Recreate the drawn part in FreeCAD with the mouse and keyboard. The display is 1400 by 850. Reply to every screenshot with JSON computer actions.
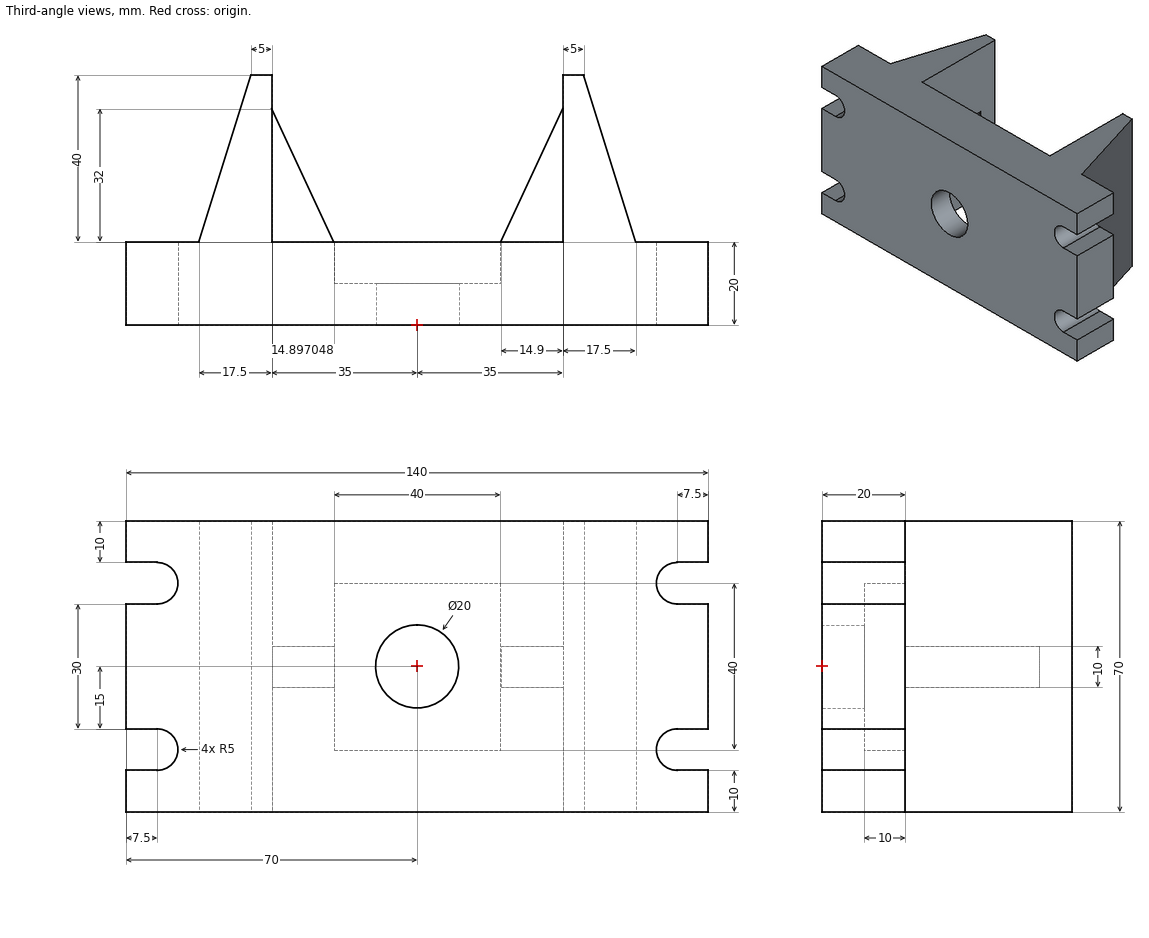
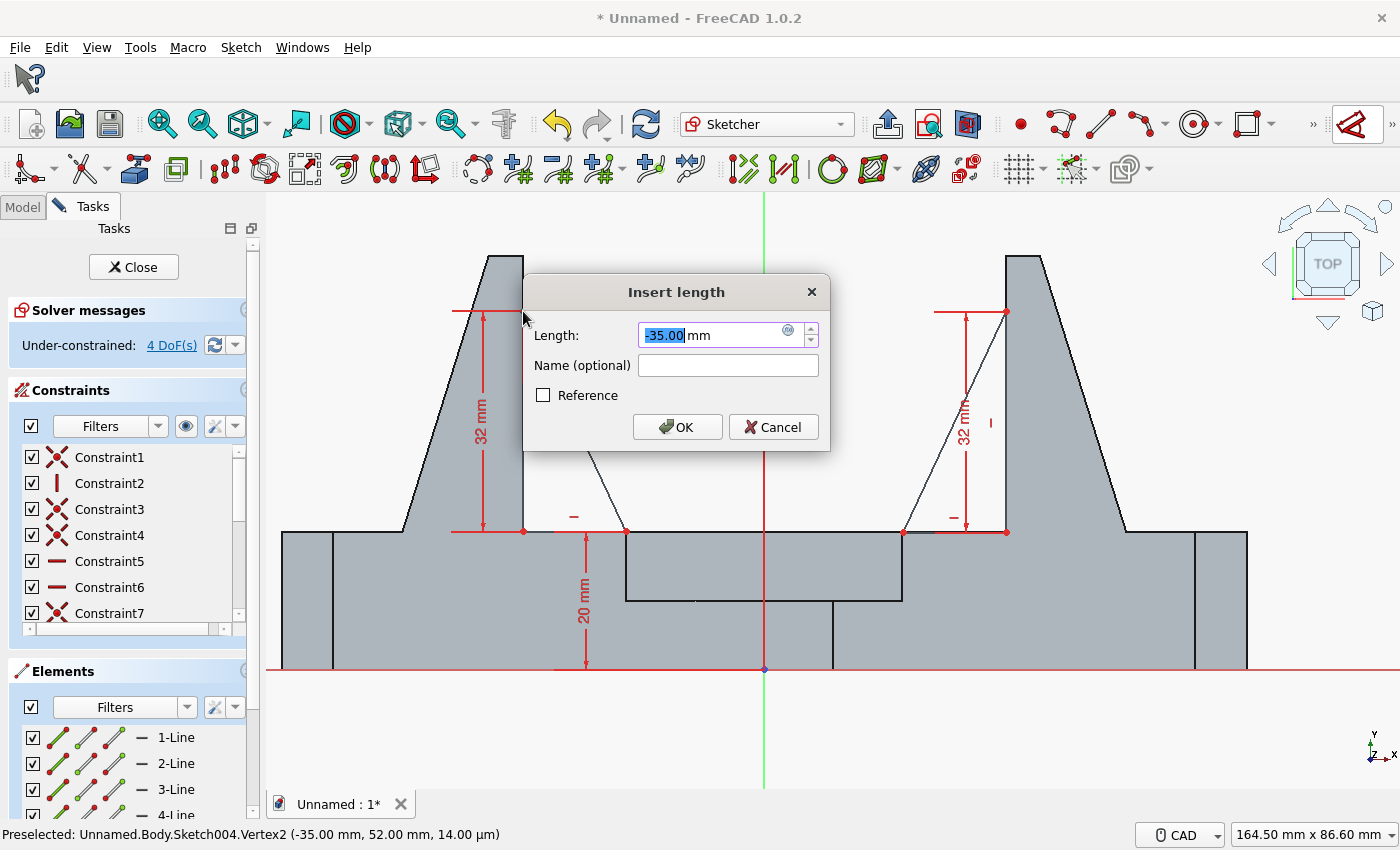
{"action": "type", "text": "-35"}
{"action": "key", "text": "Return"}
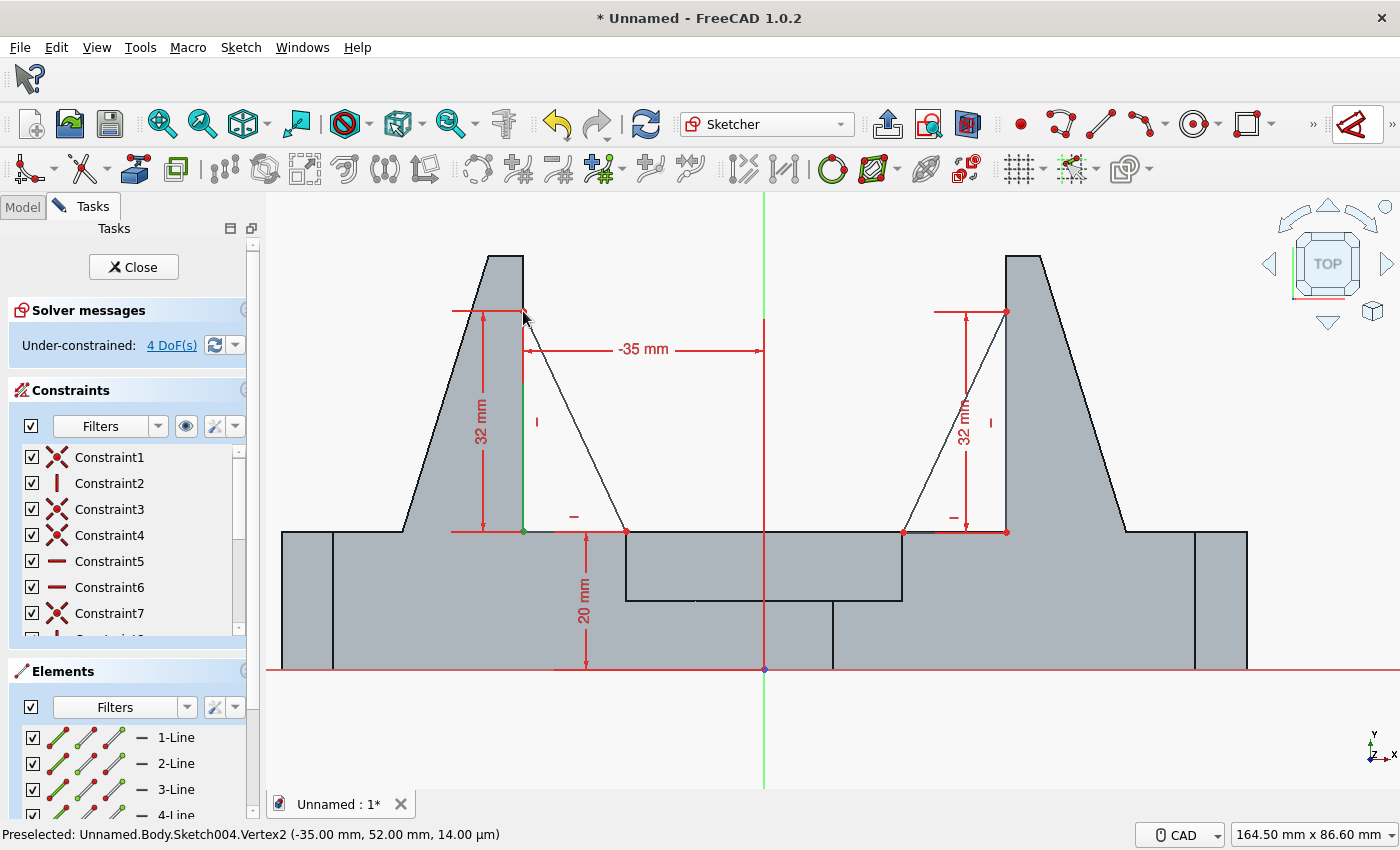
{"action": "left_click", "coordinate": [903, 533]}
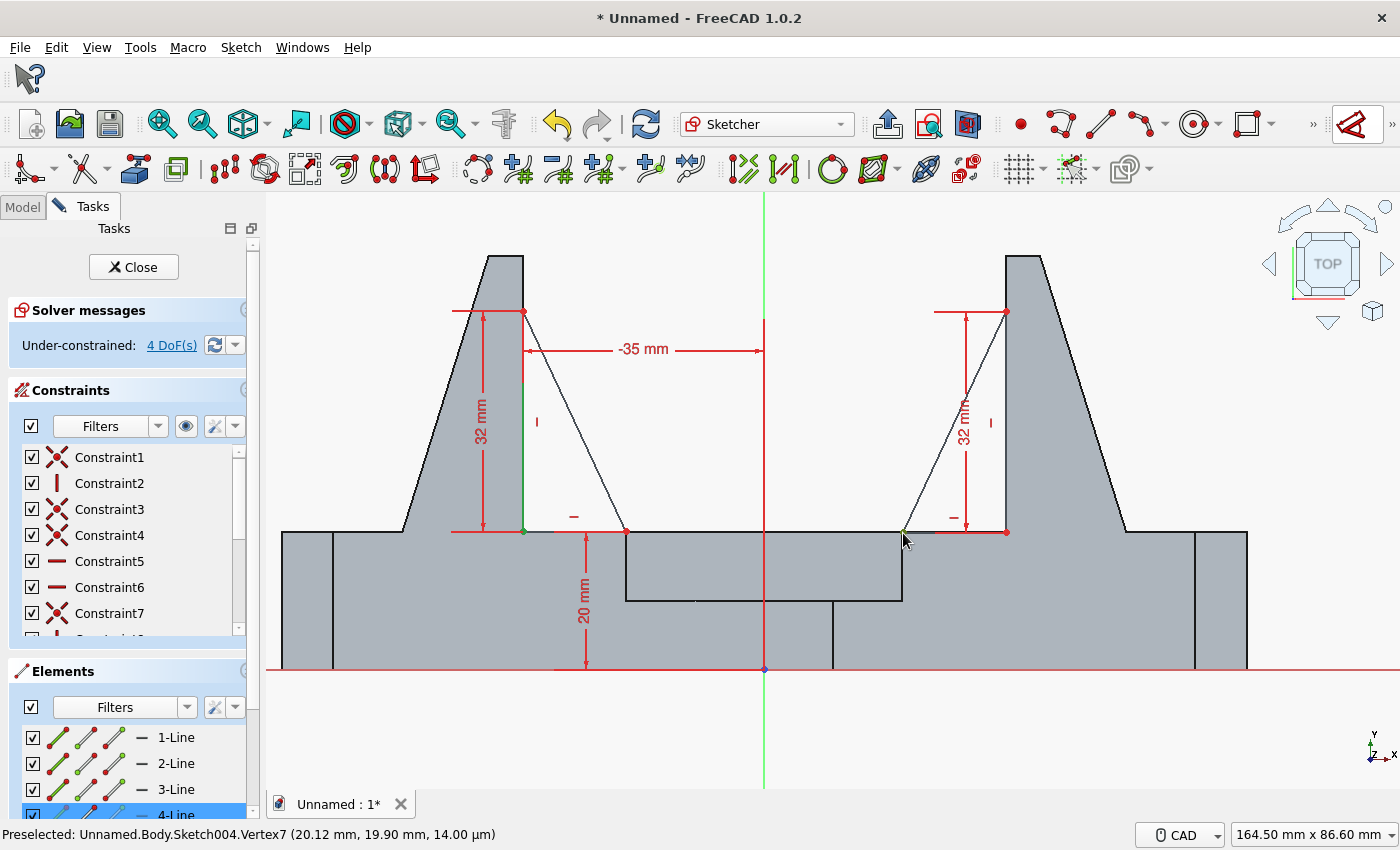
{"action": "key", "text": "i"}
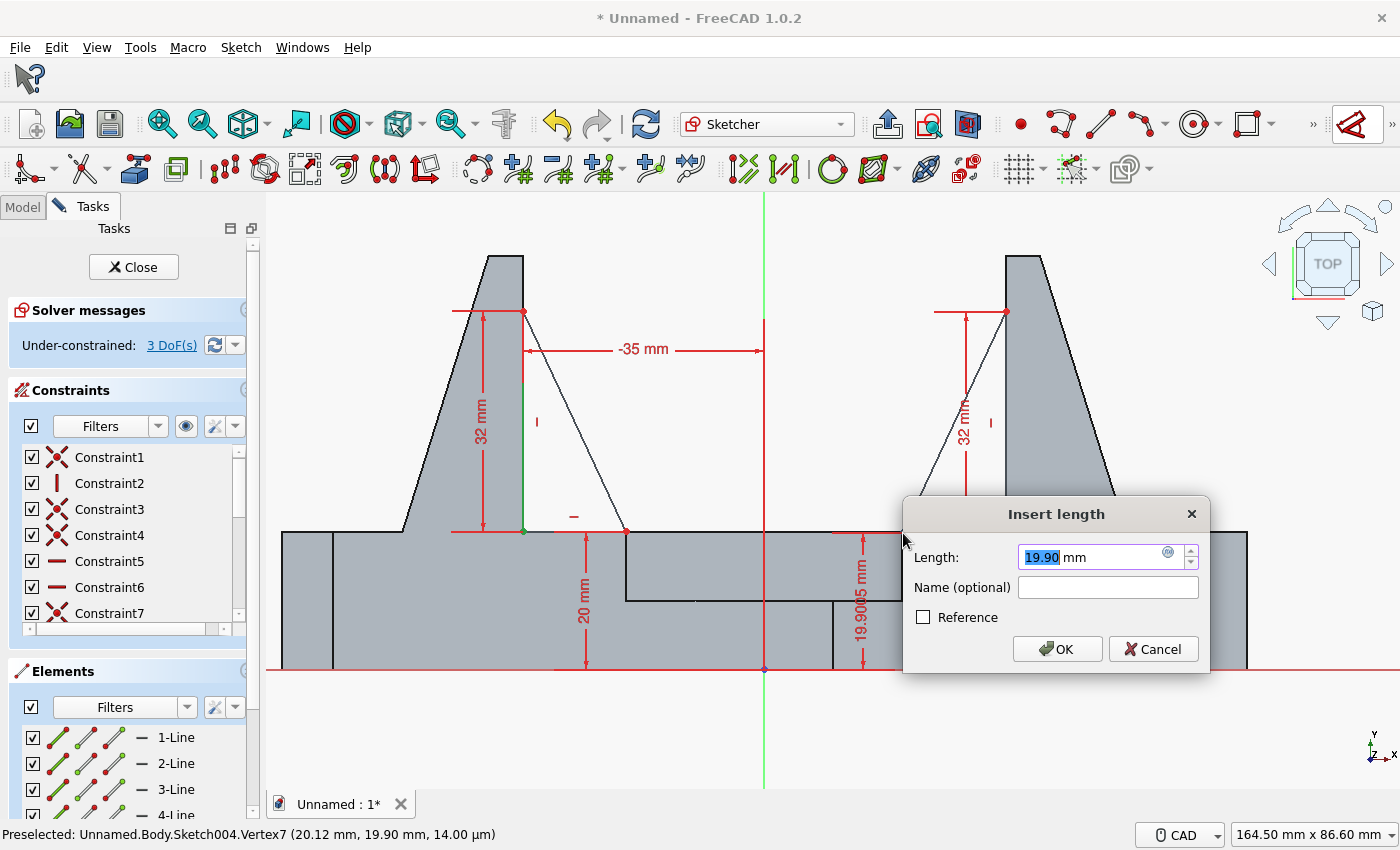
{"action": "type", "text": "20"}
{"action": "key", "text": "Return"}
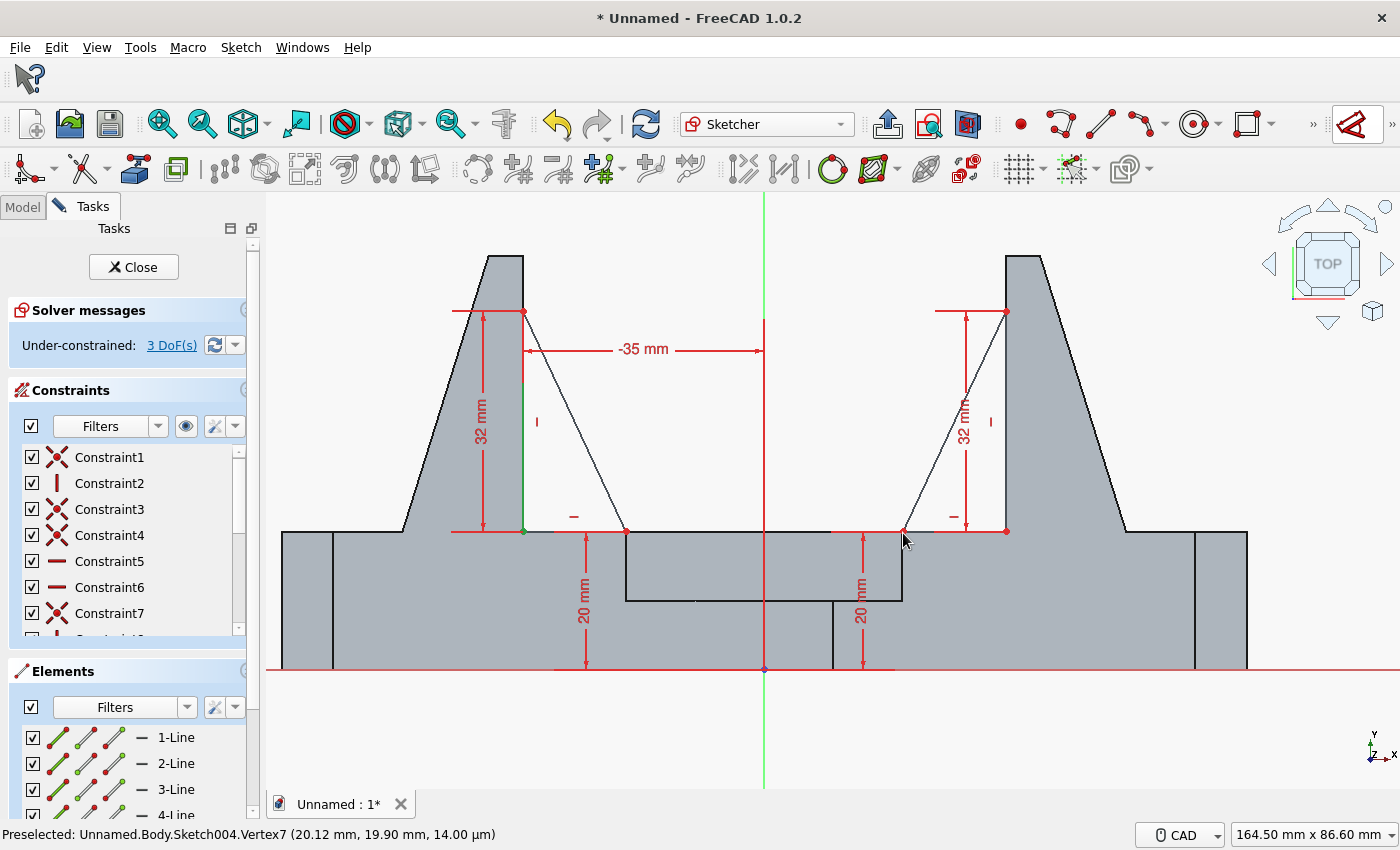
{"action": "left_click", "coordinate": [1006, 532]}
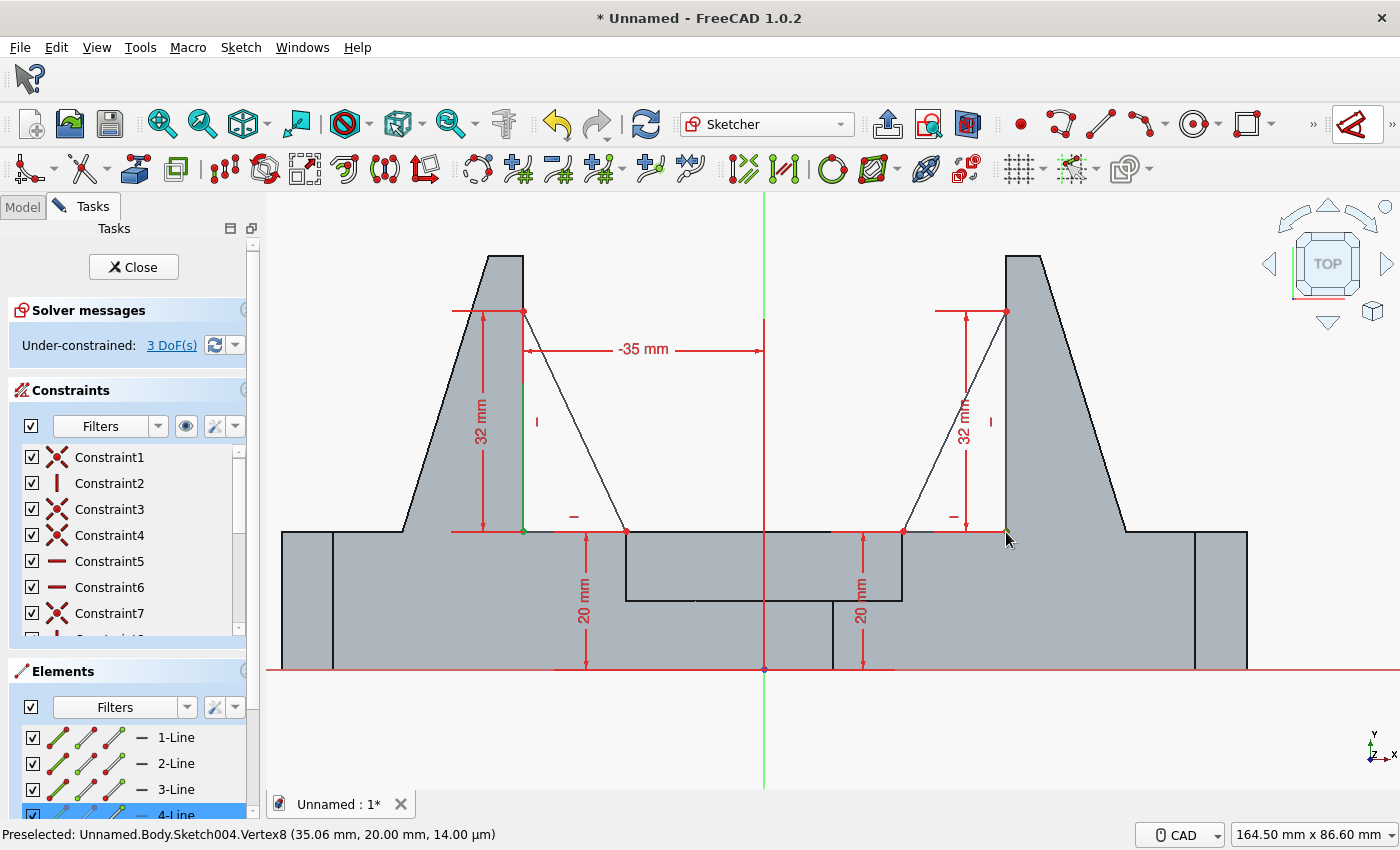
{"action": "left_click", "coordinate": [1378, 124]}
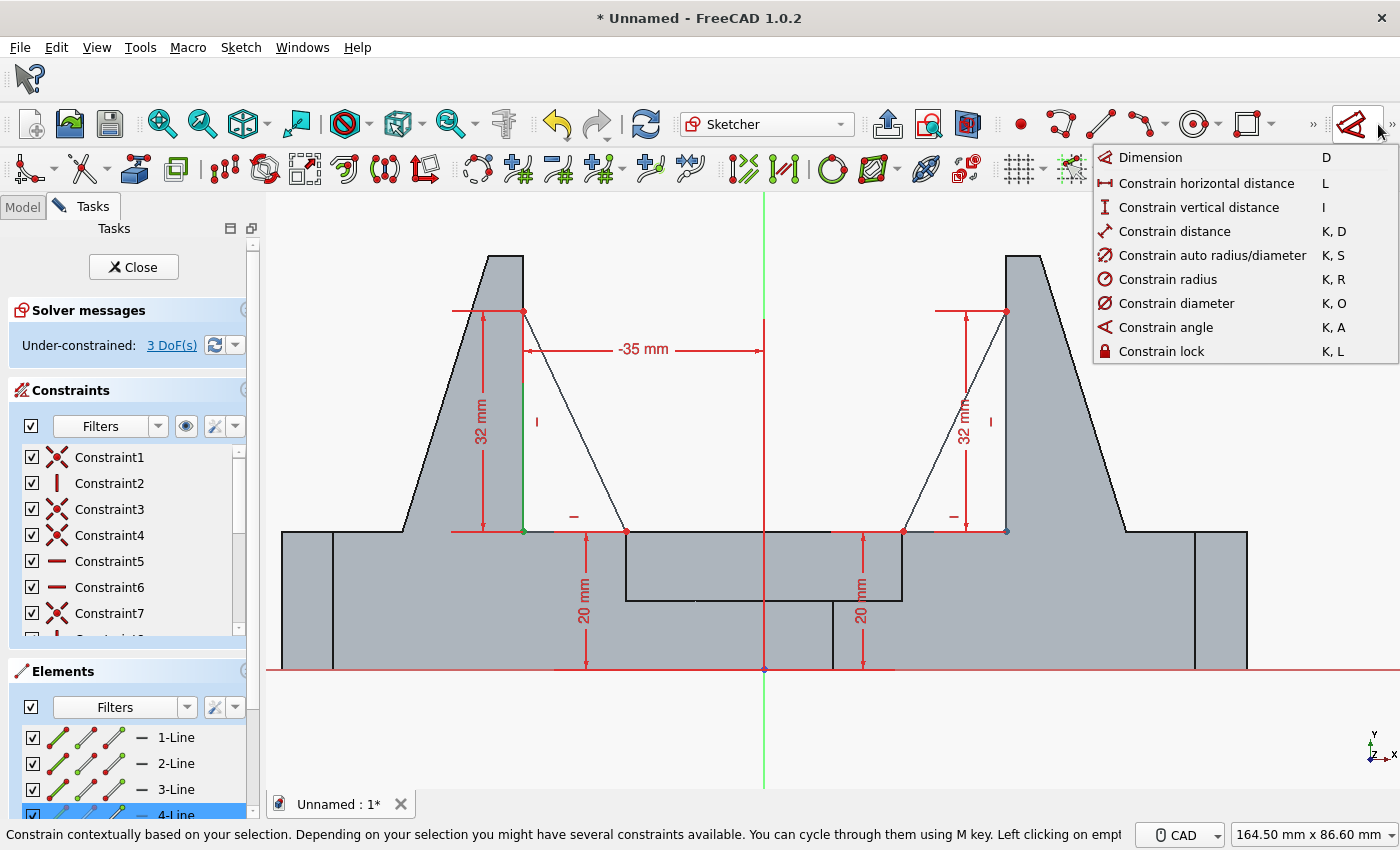
{"action": "left_click", "coordinate": [1246, 183]}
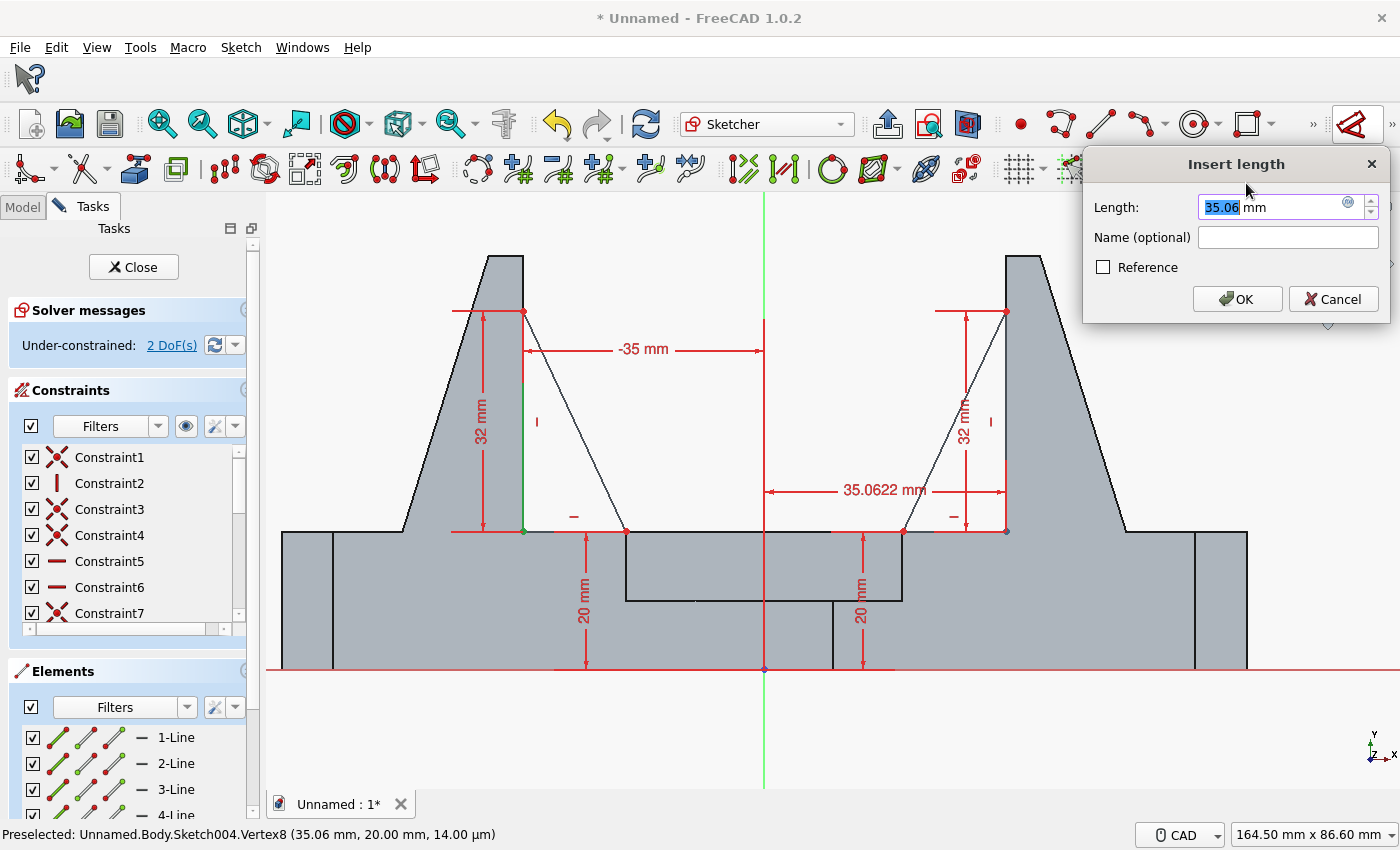
{"action": "type", "text": "35"}
{"action": "key", "text": "Return"}